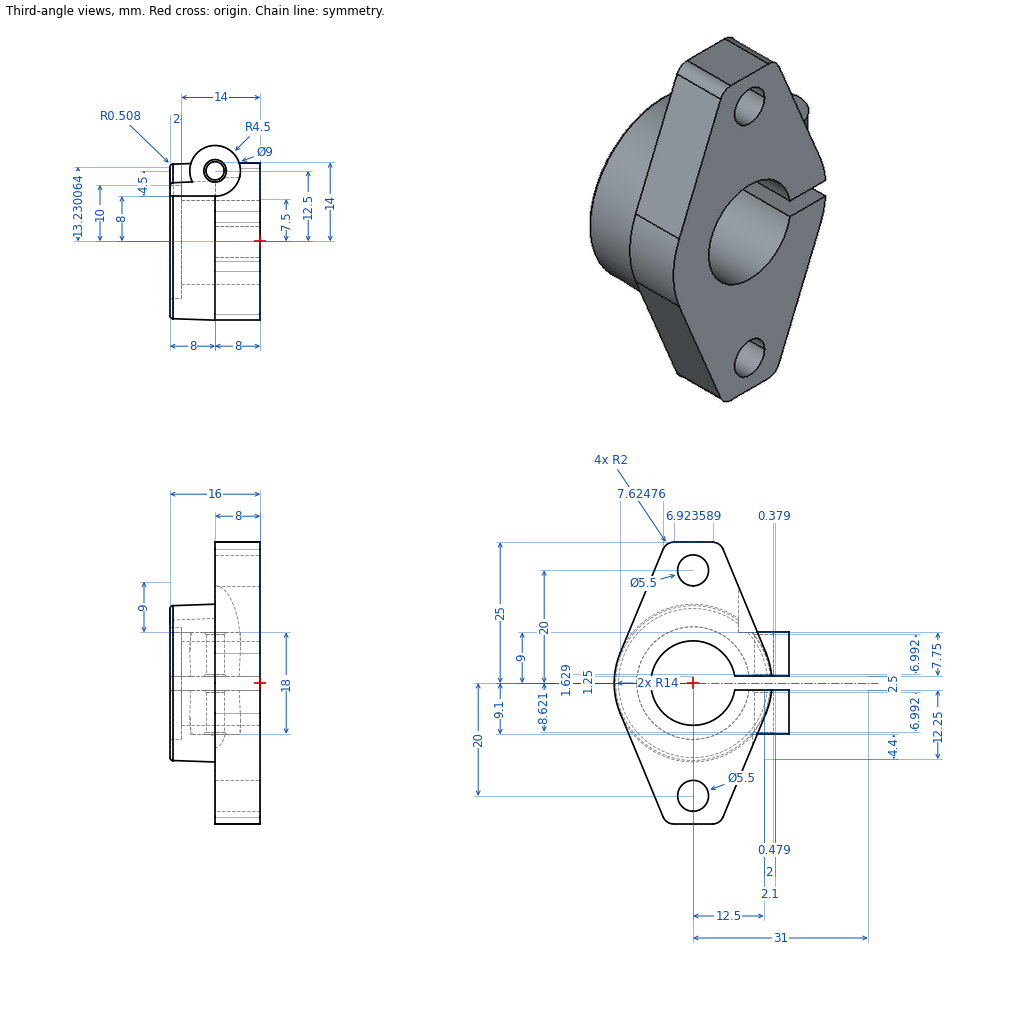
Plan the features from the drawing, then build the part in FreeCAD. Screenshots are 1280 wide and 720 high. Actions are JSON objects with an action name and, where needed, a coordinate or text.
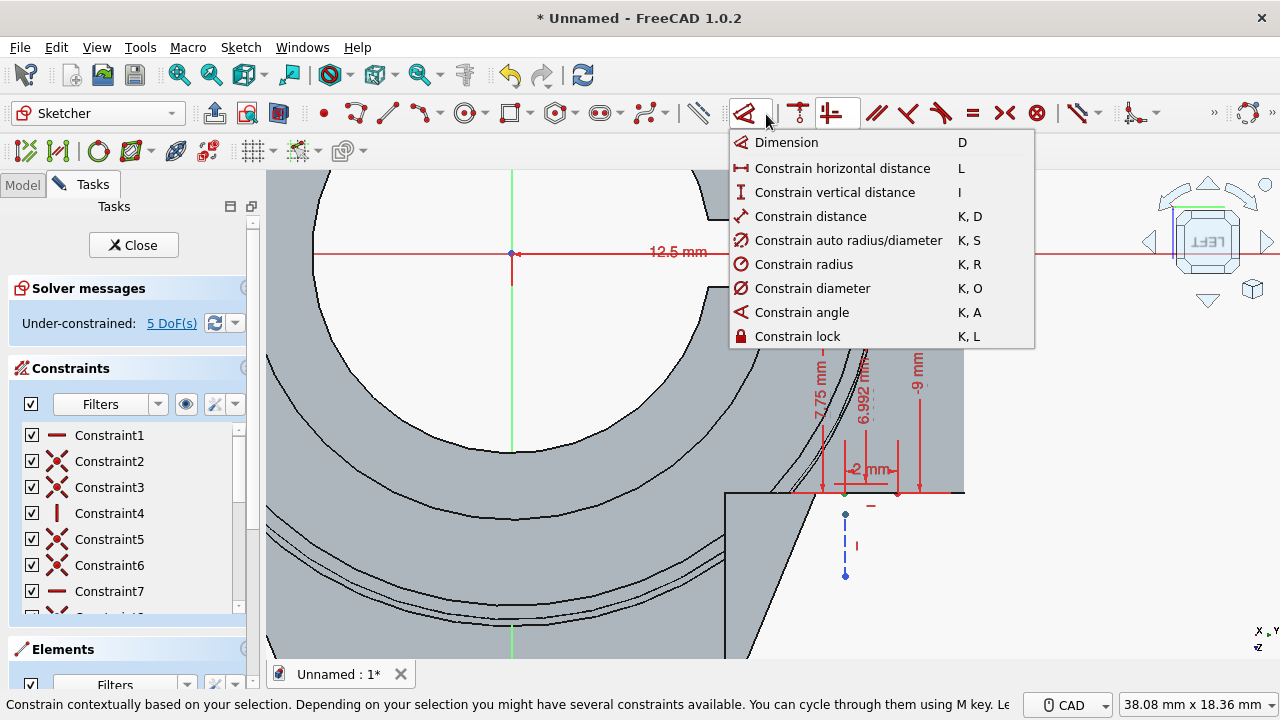
{"action": "left_click", "coordinate": [882, 168]}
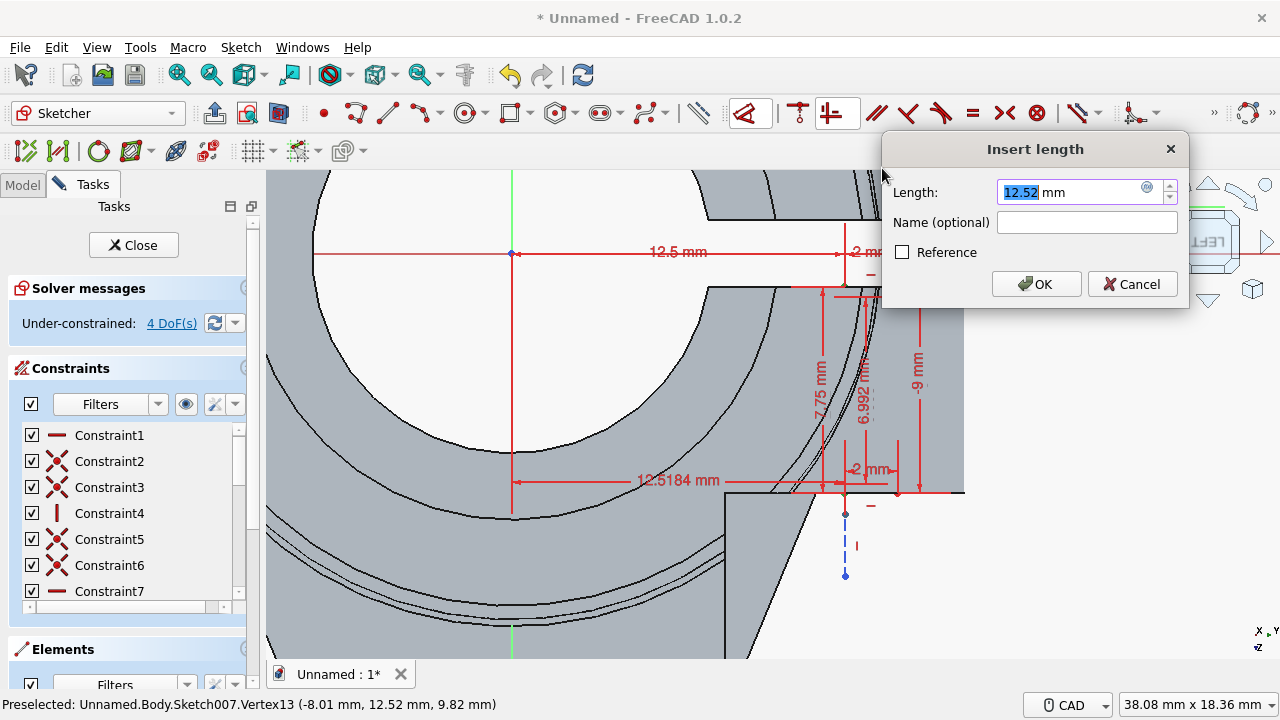
{"action": "type", "text": "12.5"}
{"action": "key", "text": "Return"}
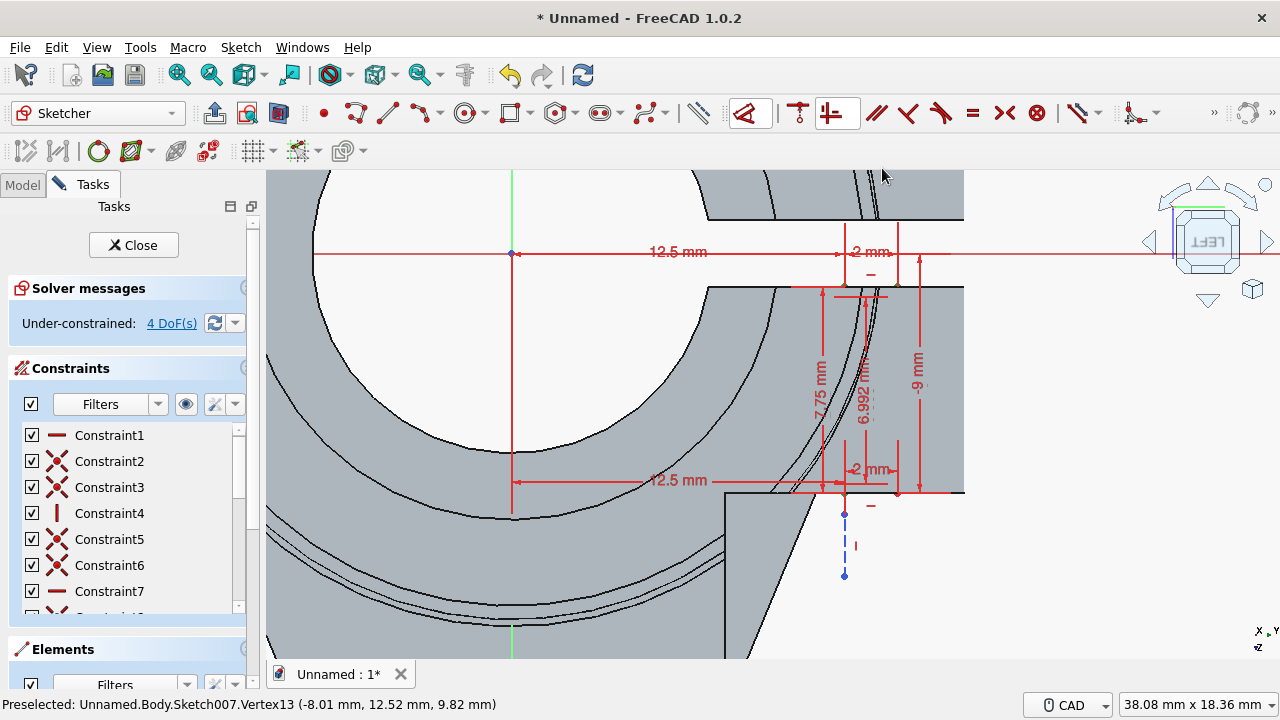
{"action": "left_click", "coordinate": [887, 297]}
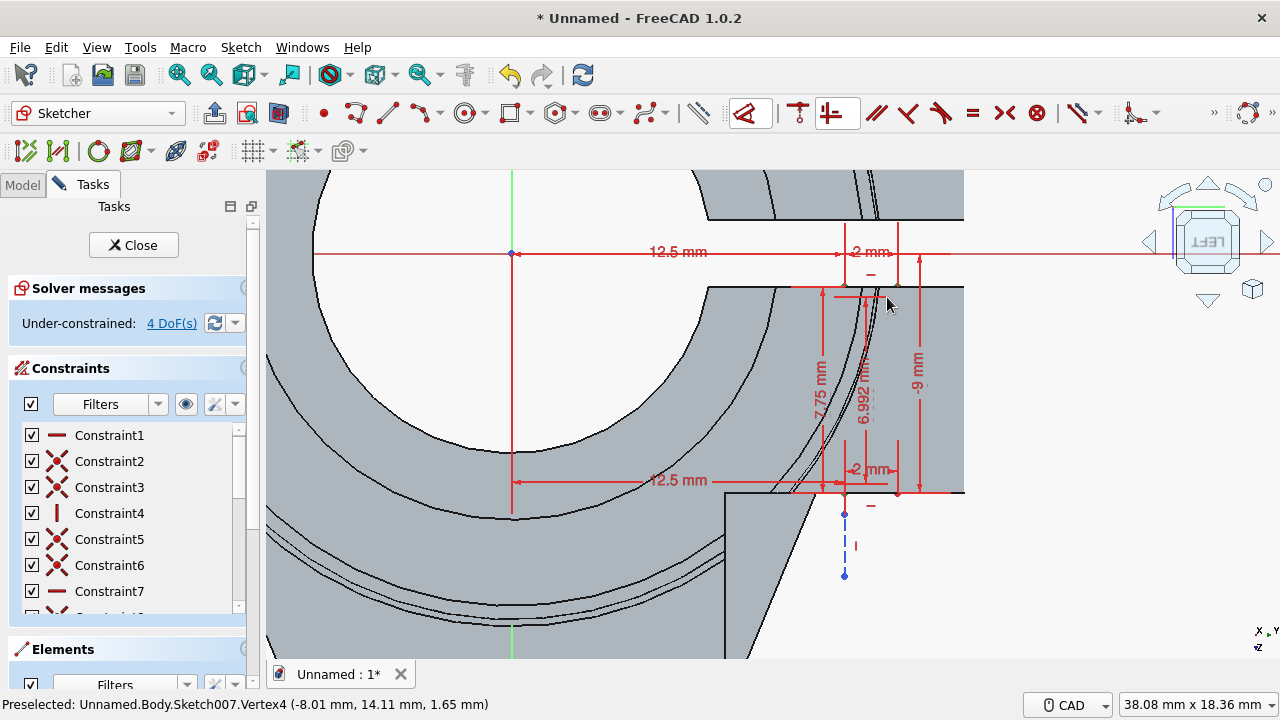
{"action": "left_click", "coordinate": [766, 114]}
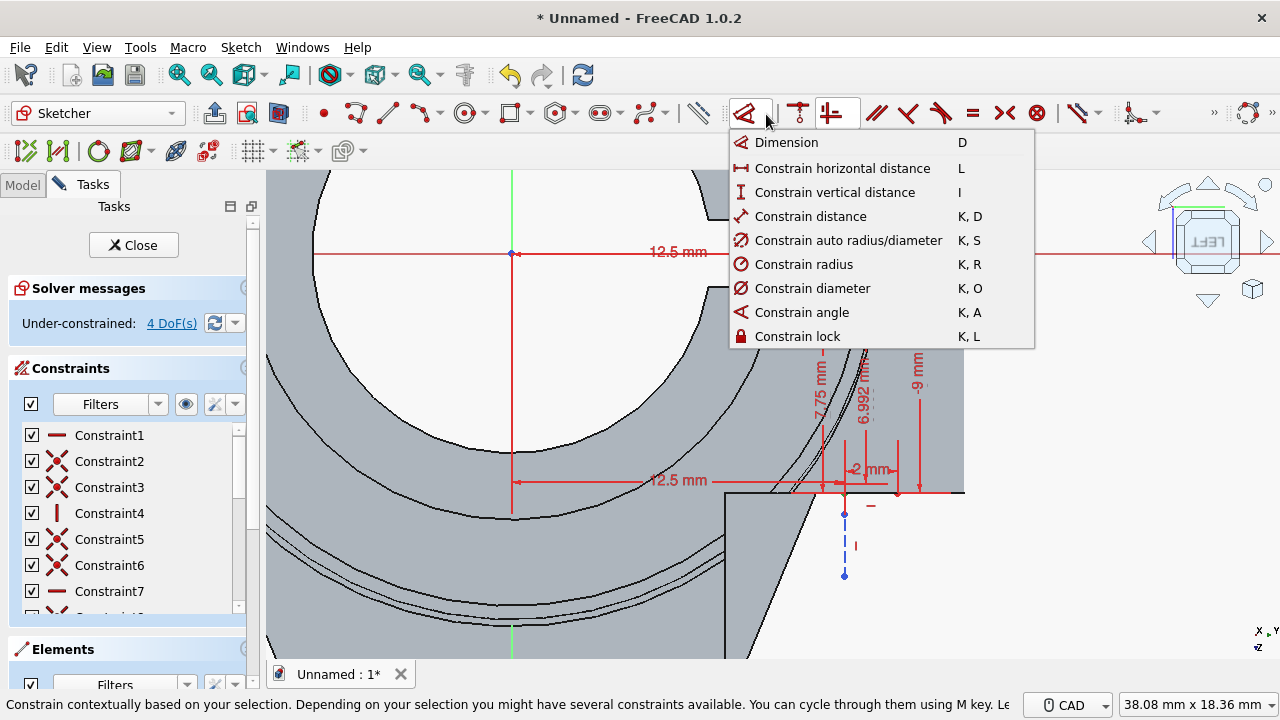
{"action": "left_click", "coordinate": [882, 192]}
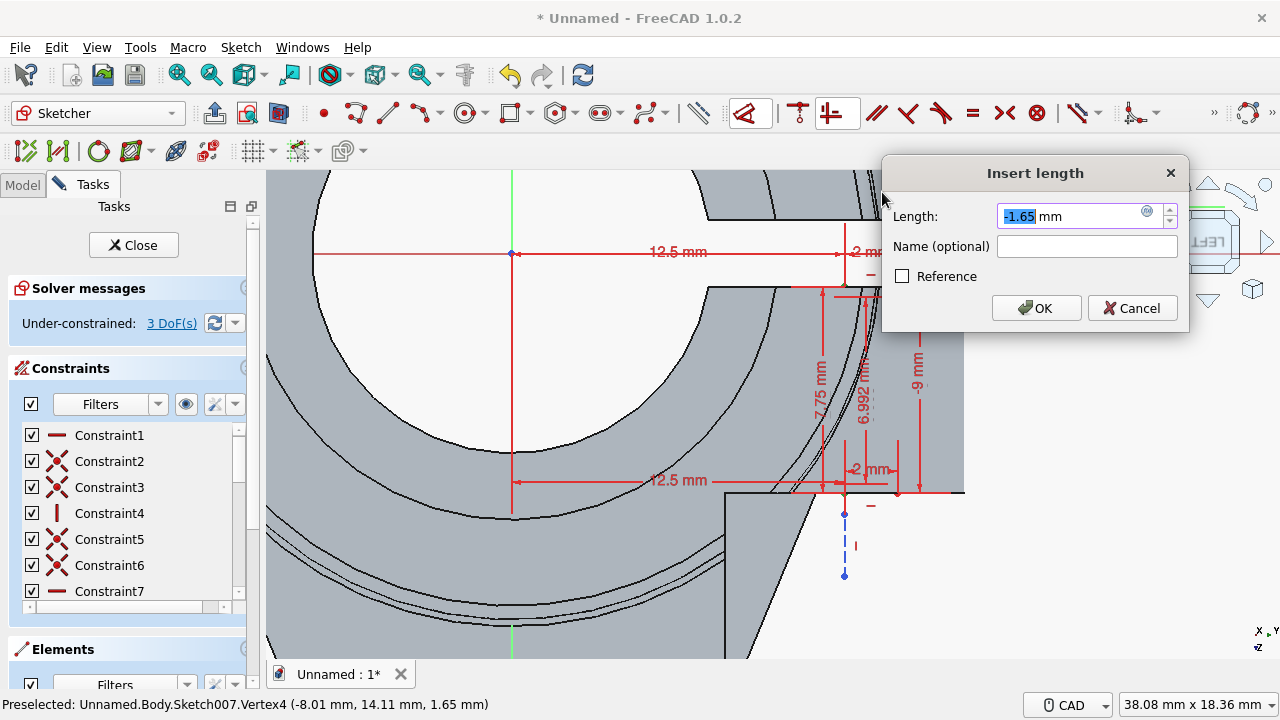
{"action": "type", "text": "-1.629"}
{"action": "key", "text": "Return"}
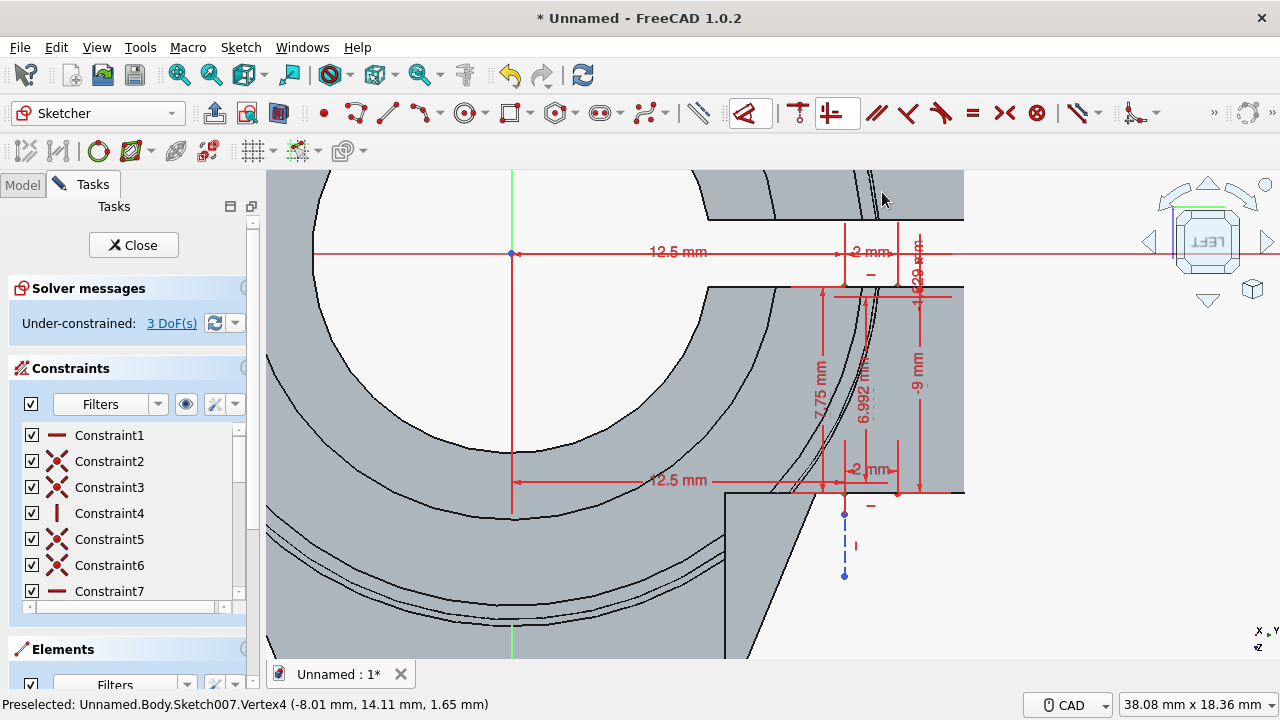
{"action": "scroll", "coordinate": [892, 293], "scroll_direction": "up", "scroll_amount": 7}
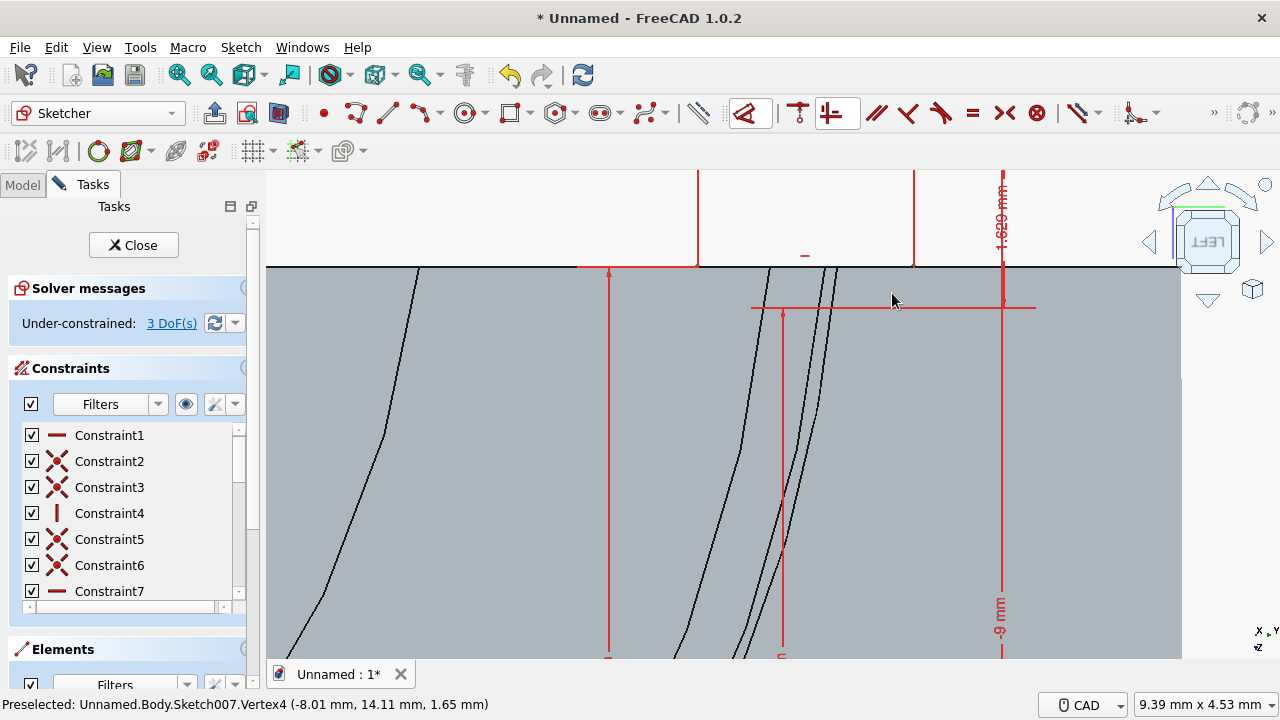
{"action": "left_click", "coordinate": [888, 292]}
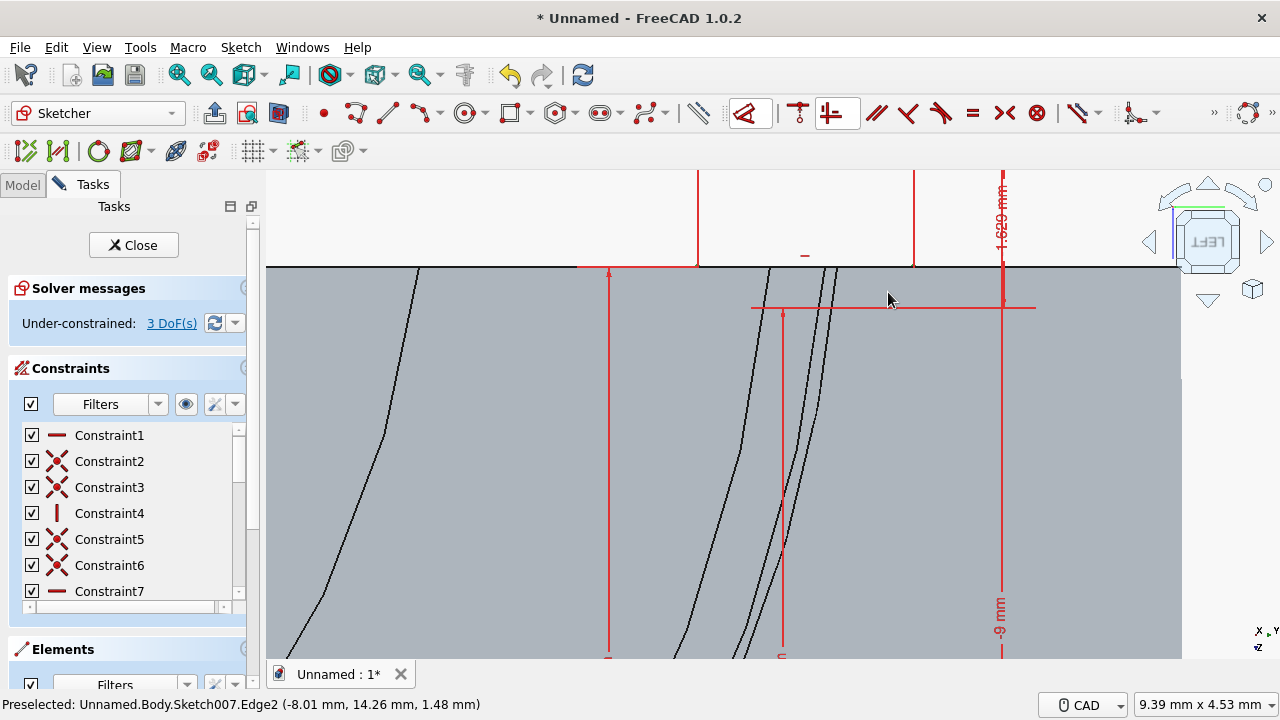
{"action": "left_click", "coordinate": [766, 114]}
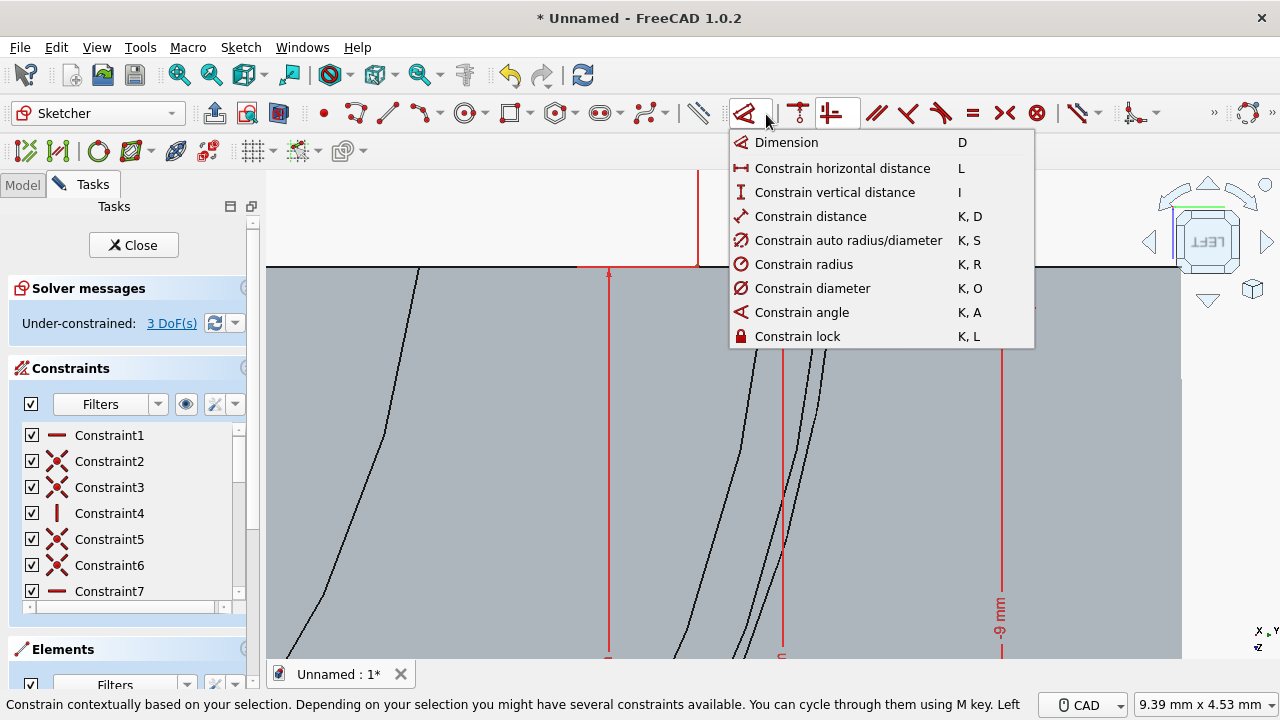
{"action": "left_click", "coordinate": [882, 168]}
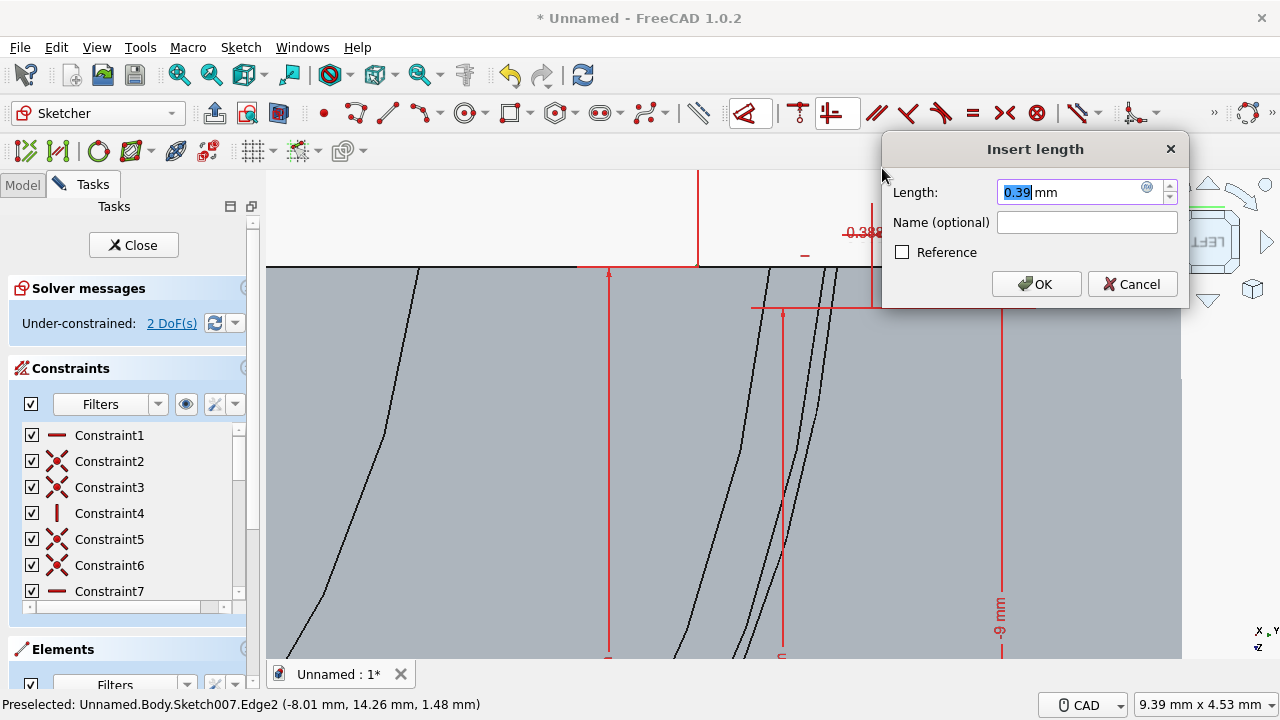
{"action": "type", "text": "0.379"}
{"action": "key", "text": "Return"}